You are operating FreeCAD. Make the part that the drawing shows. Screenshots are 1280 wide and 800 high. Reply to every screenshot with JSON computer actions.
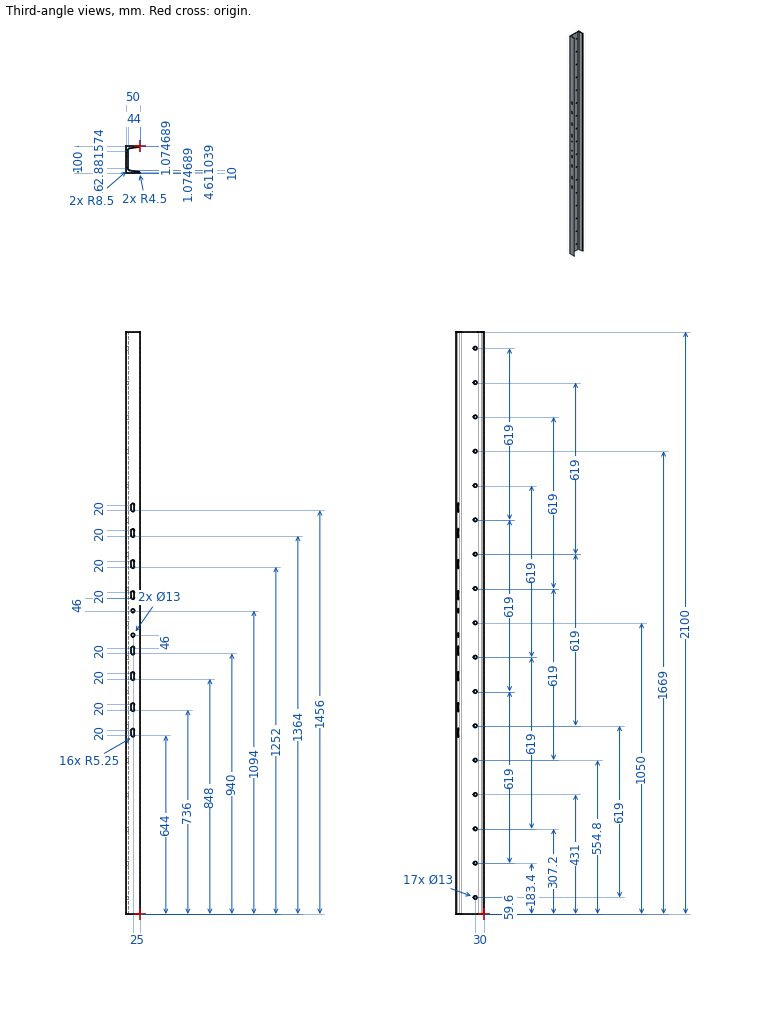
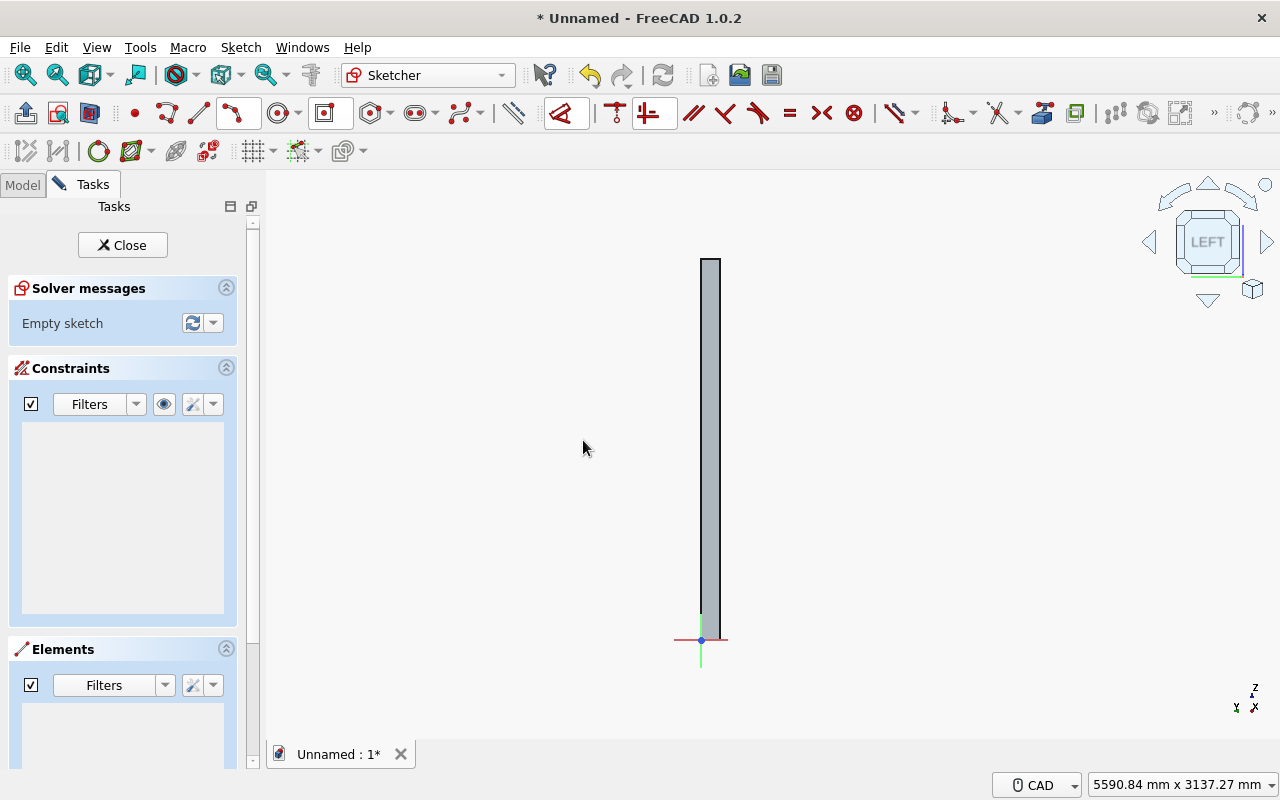
{"action": "left_click", "coordinate": [278, 114]}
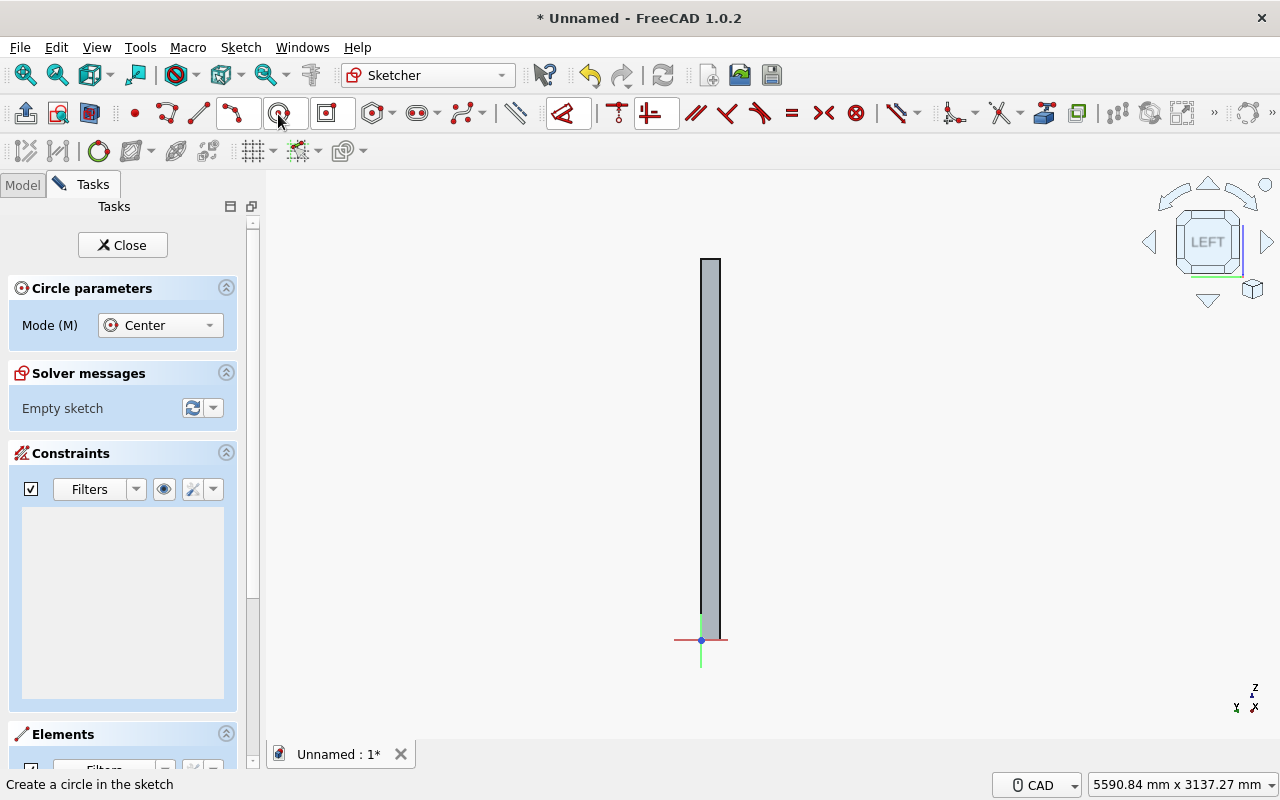
{"action": "scroll", "coordinate": [707, 630], "scroll_direction": "up", "scroll_amount": 15}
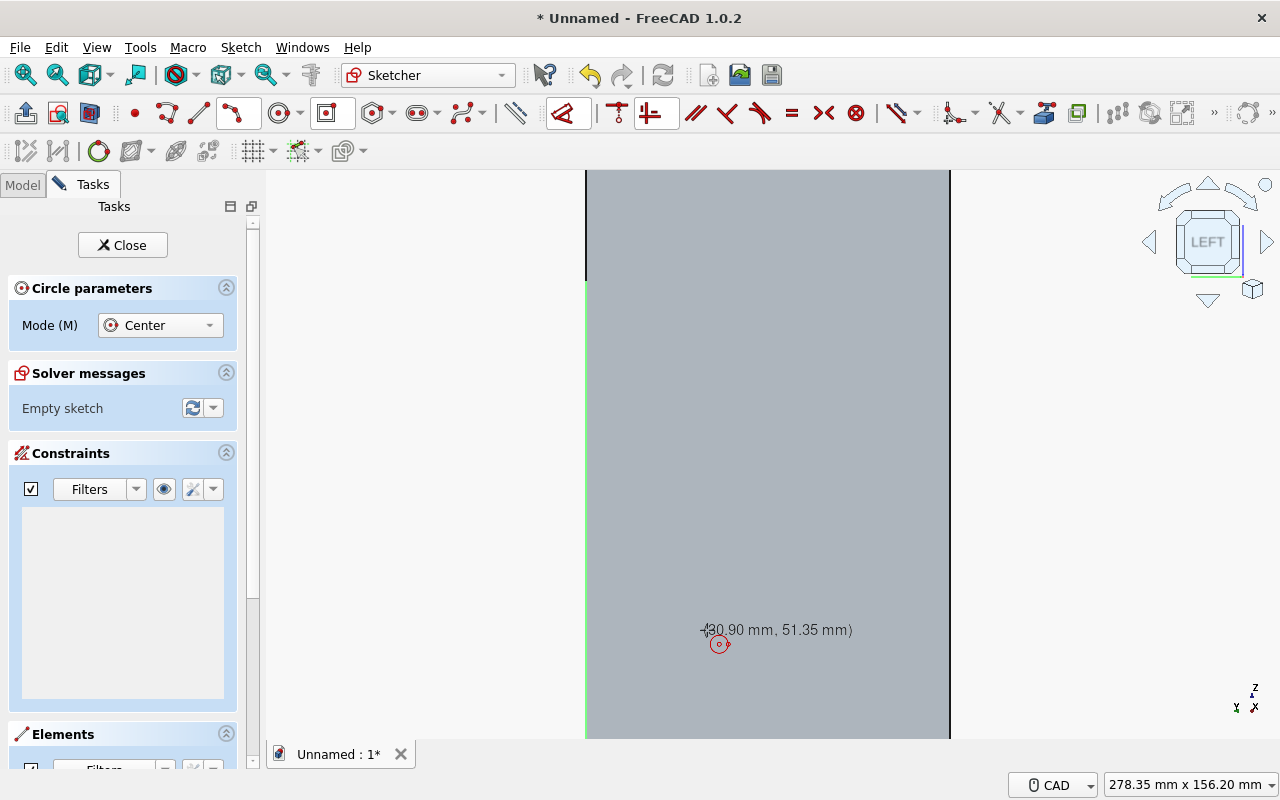
{"action": "scroll", "coordinate": [707, 631], "scroll_direction": "down", "scroll_amount": 15}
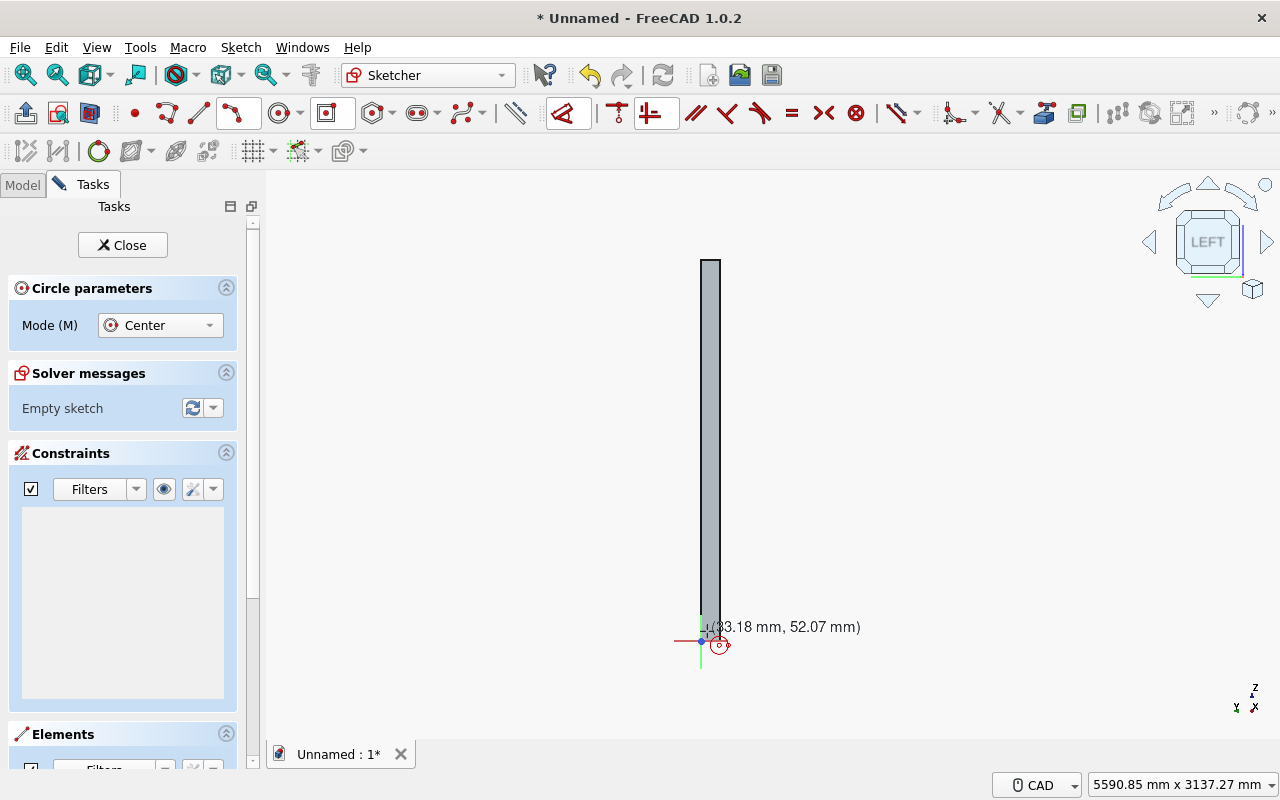
{"action": "scroll", "coordinate": [707, 630], "scroll_direction": "up", "scroll_amount": 6}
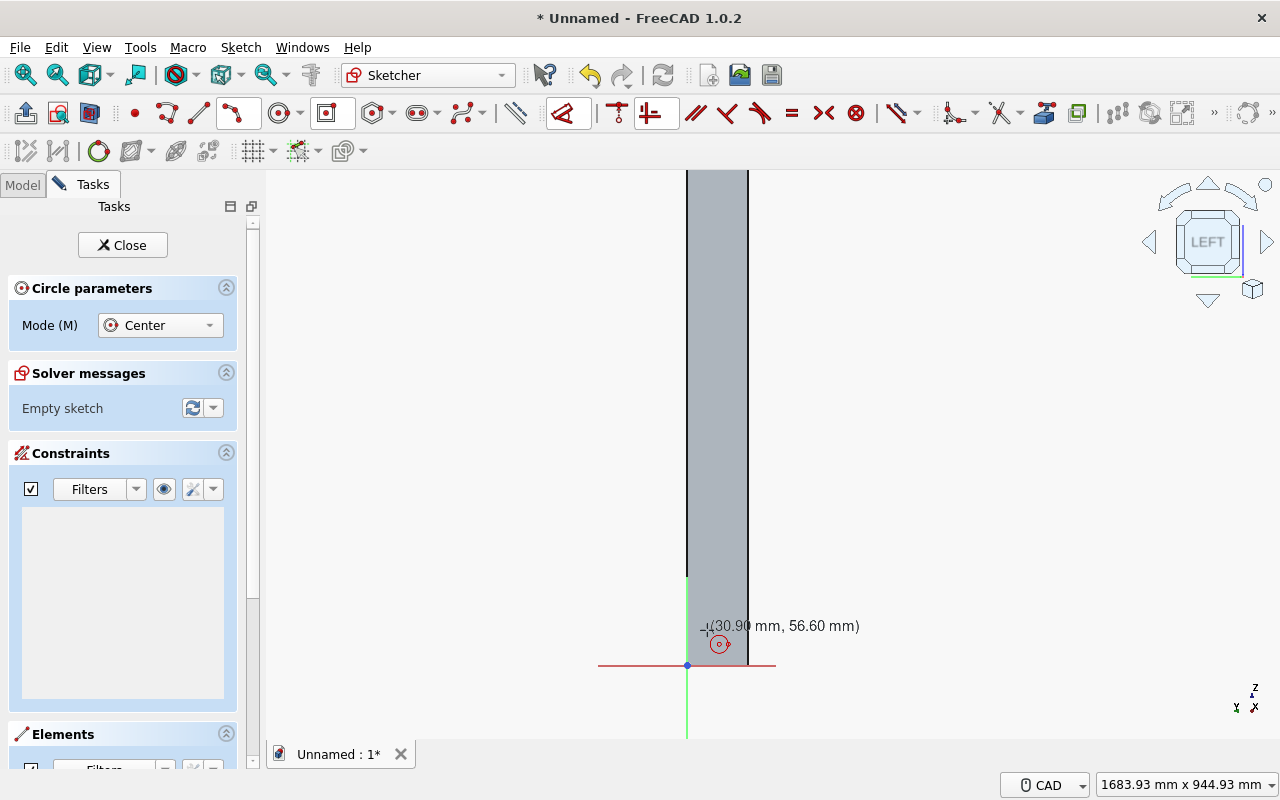
{"action": "left_click", "coordinate": [705, 630]}
{"action": "mouse_move", "coordinate": [708, 627]}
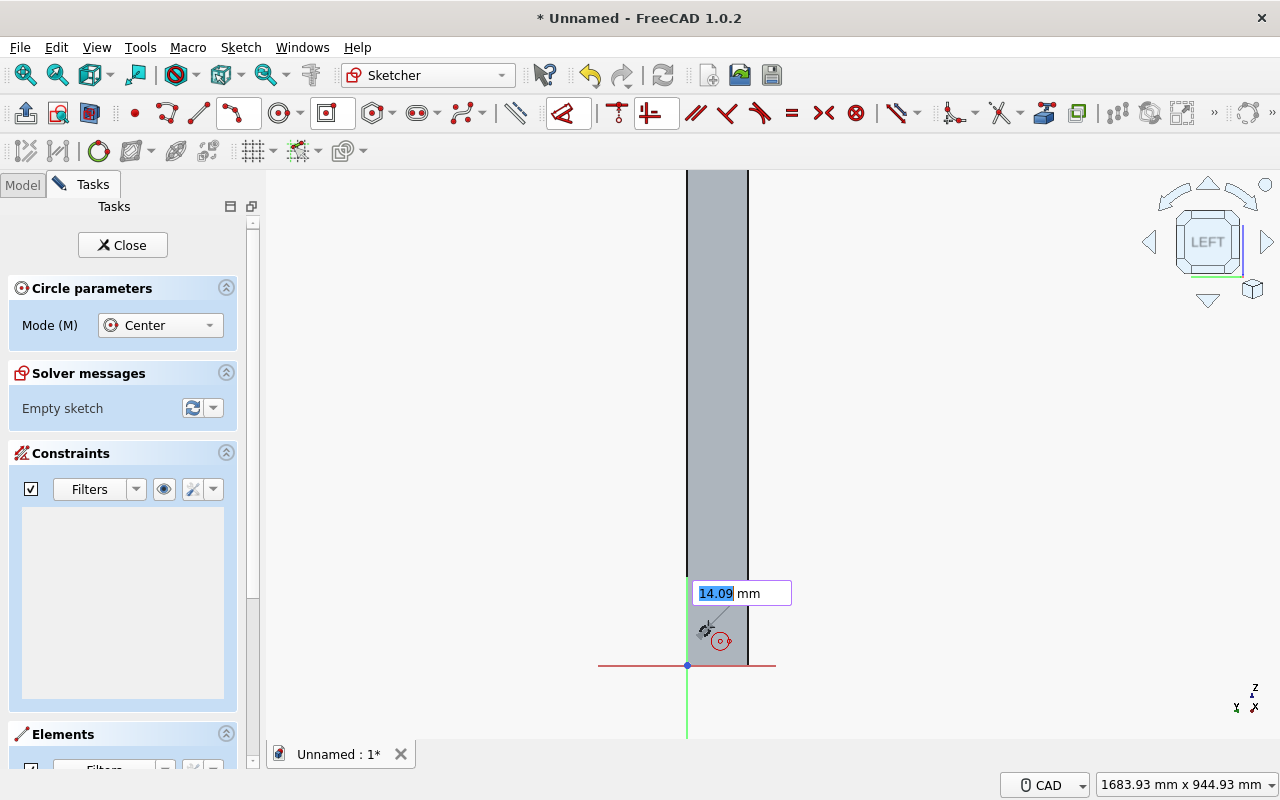
{"action": "type", "text": "13"}
{"action": "key", "text": "Return"}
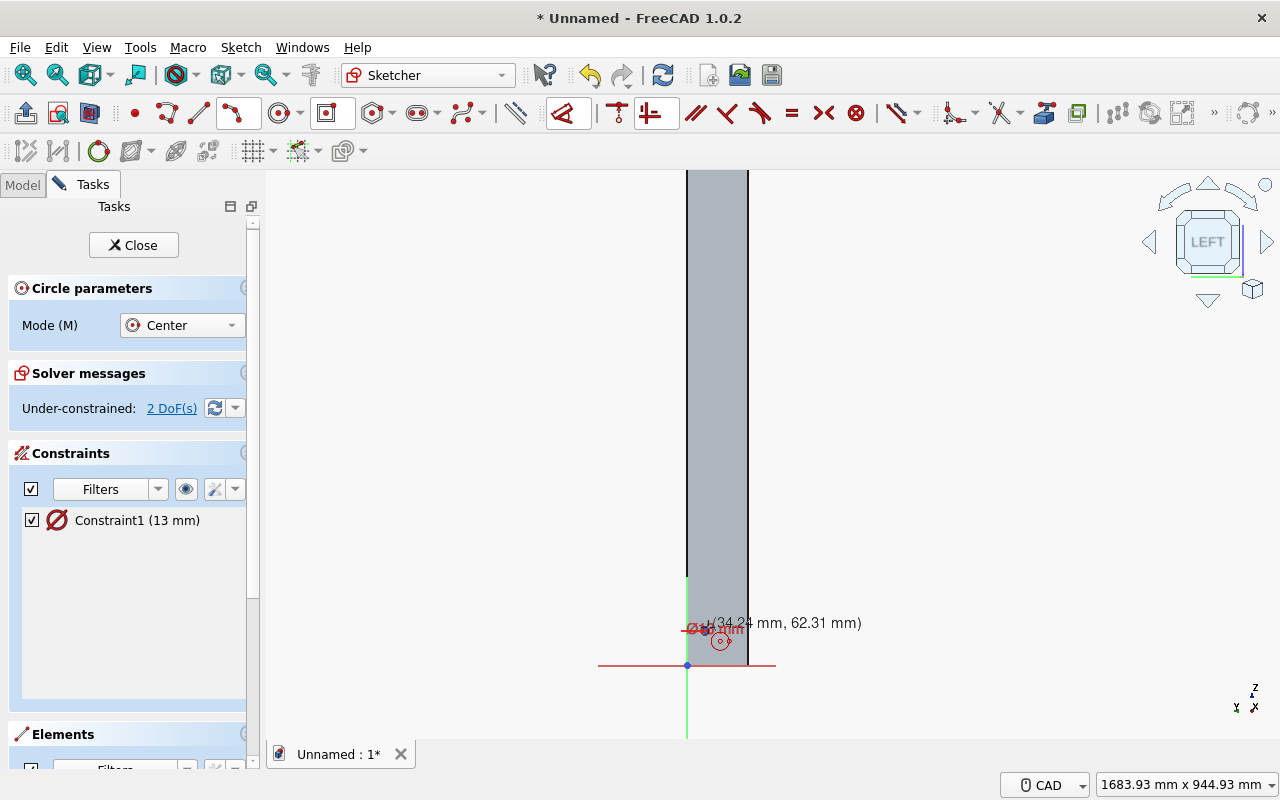
{"action": "scroll", "coordinate": [705, 555], "scroll_direction": "up", "scroll_amount": 9}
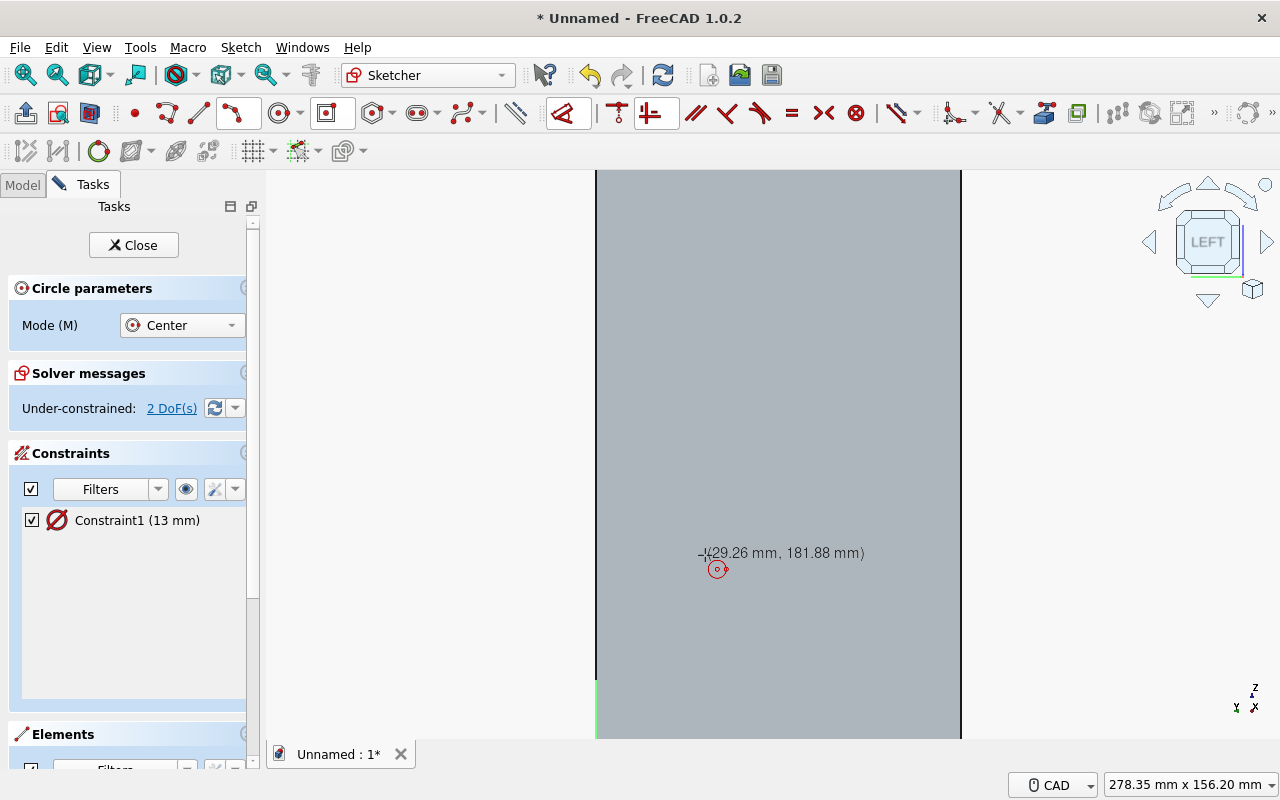
{"action": "scroll", "coordinate": [707, 610], "scroll_direction": "down", "scroll_amount": 15}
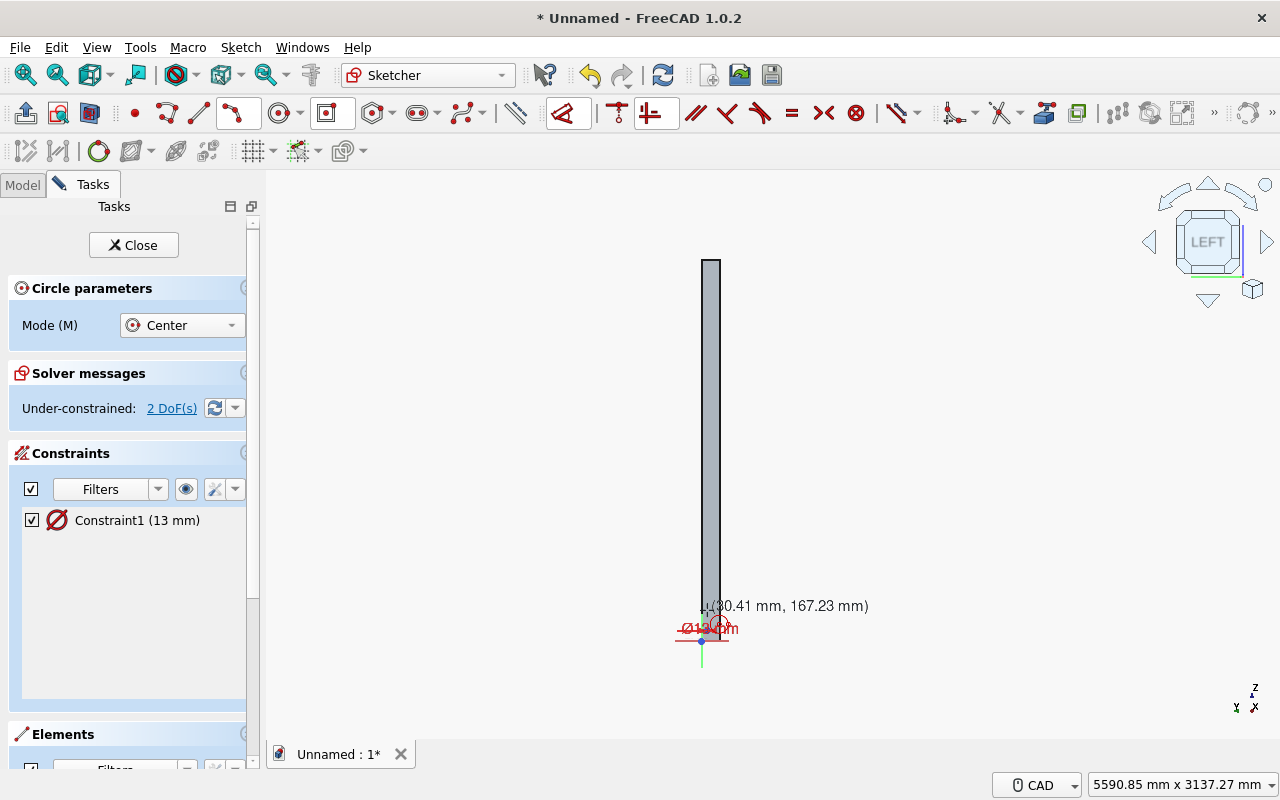
{"action": "scroll", "coordinate": [707, 608], "scroll_direction": "up", "scroll_amount": 6}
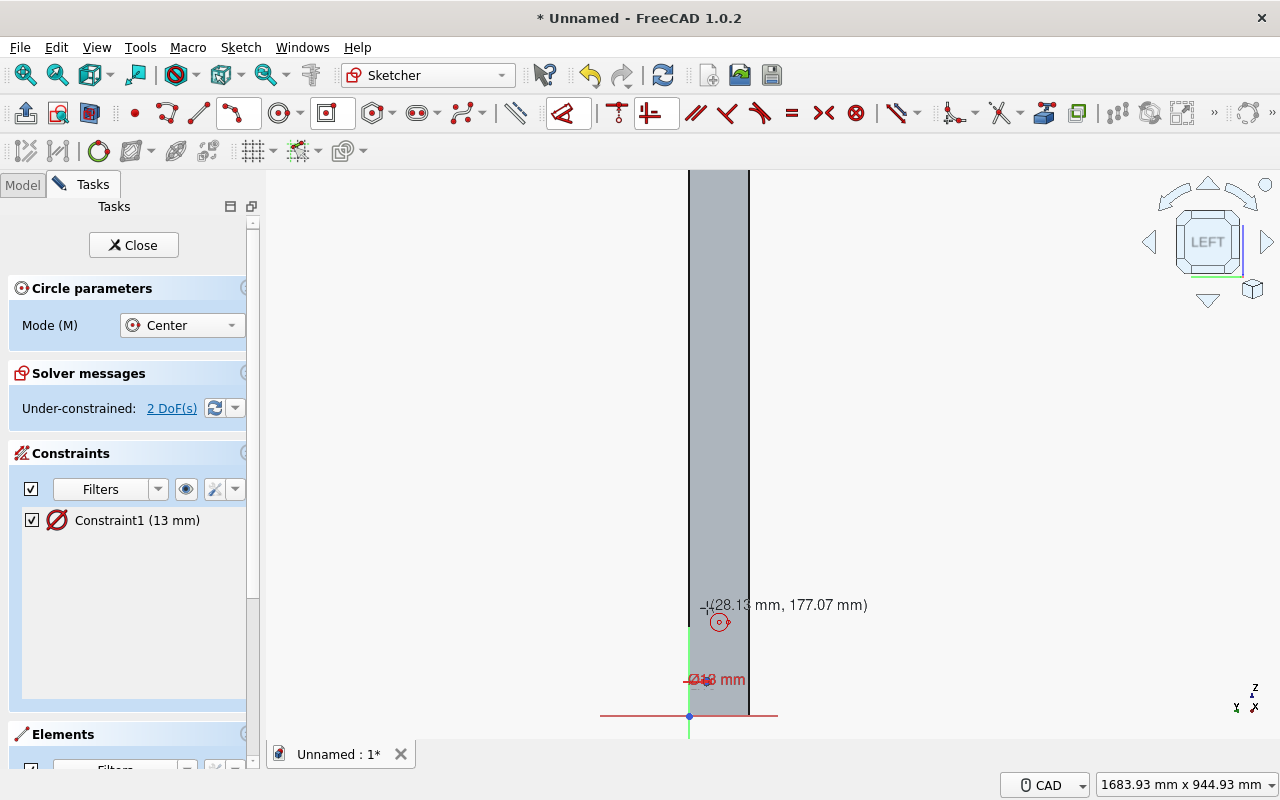
{"action": "left_click", "coordinate": [707, 606]}
{"action": "mouse_move", "coordinate": [710, 603]}